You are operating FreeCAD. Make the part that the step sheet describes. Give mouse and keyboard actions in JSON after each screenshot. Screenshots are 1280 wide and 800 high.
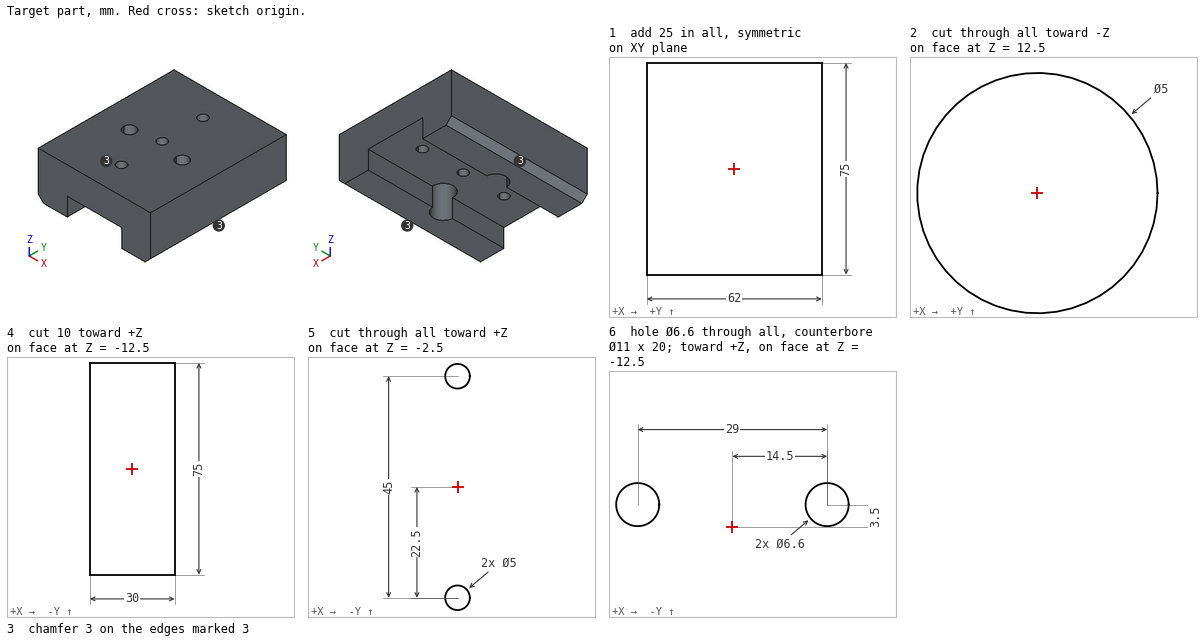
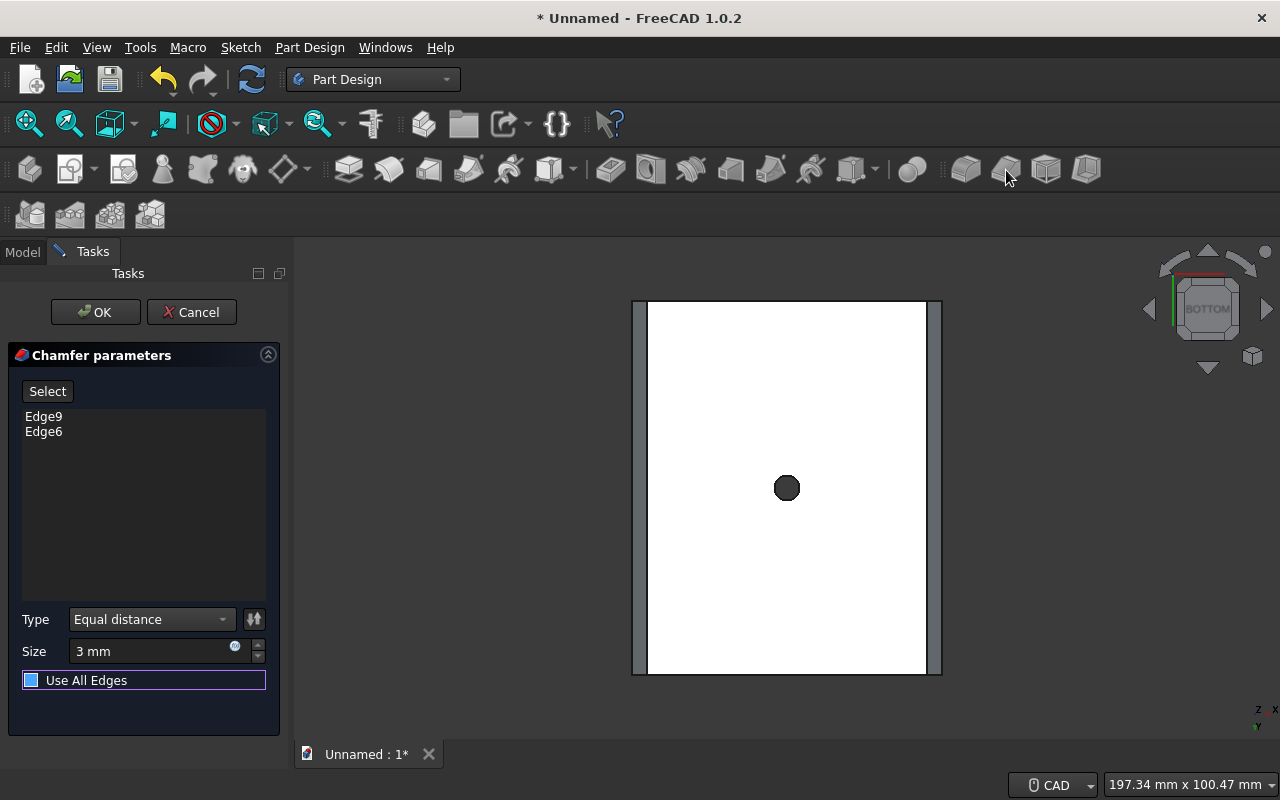
{"action": "left_click", "coordinate": [96, 312]}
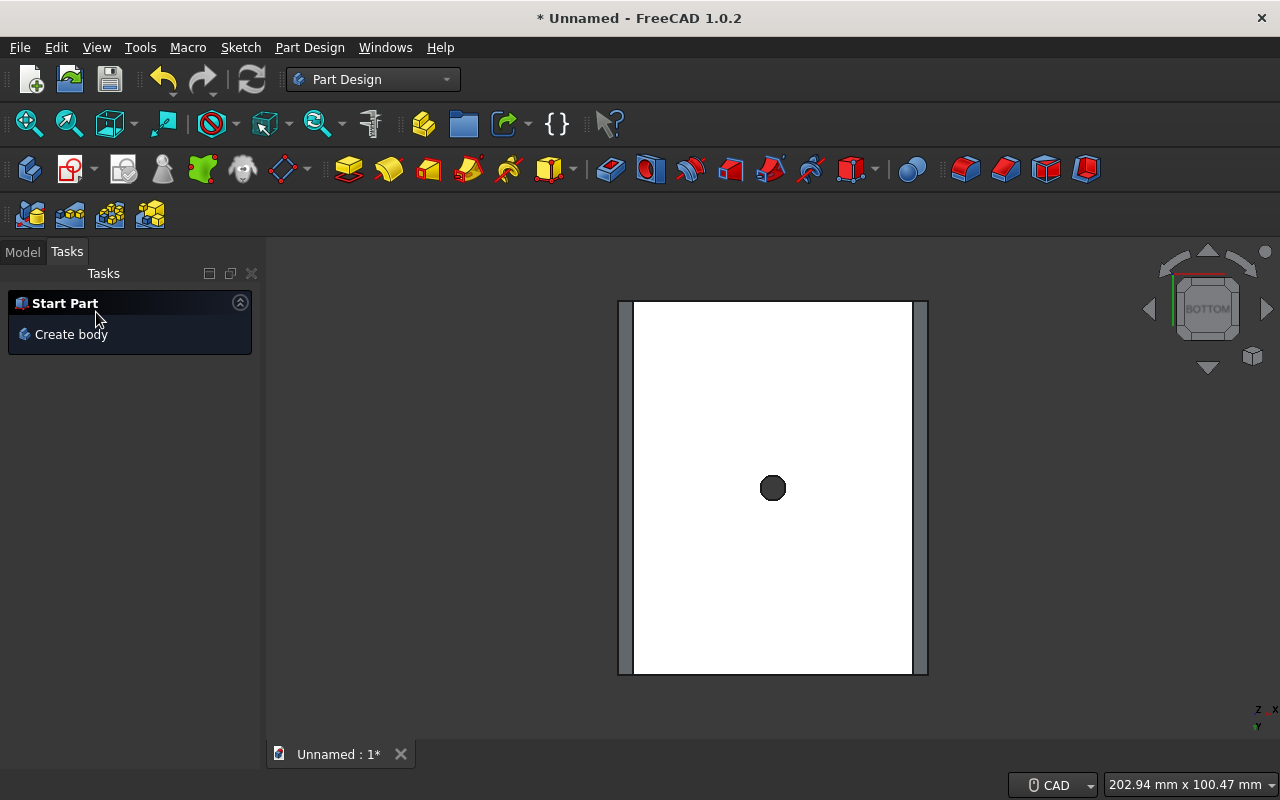
{"action": "left_click", "coordinate": [813, 380]}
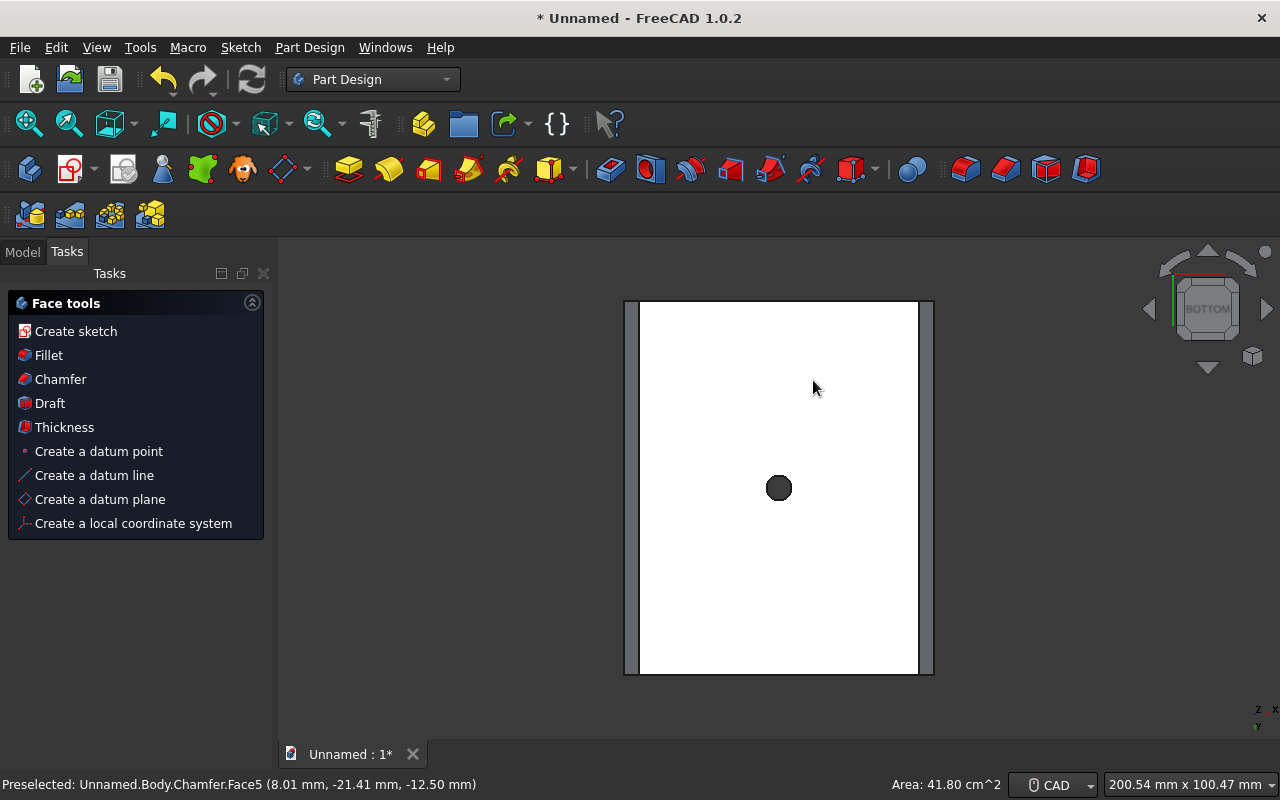
{"action": "left_click", "coordinate": [70, 170]}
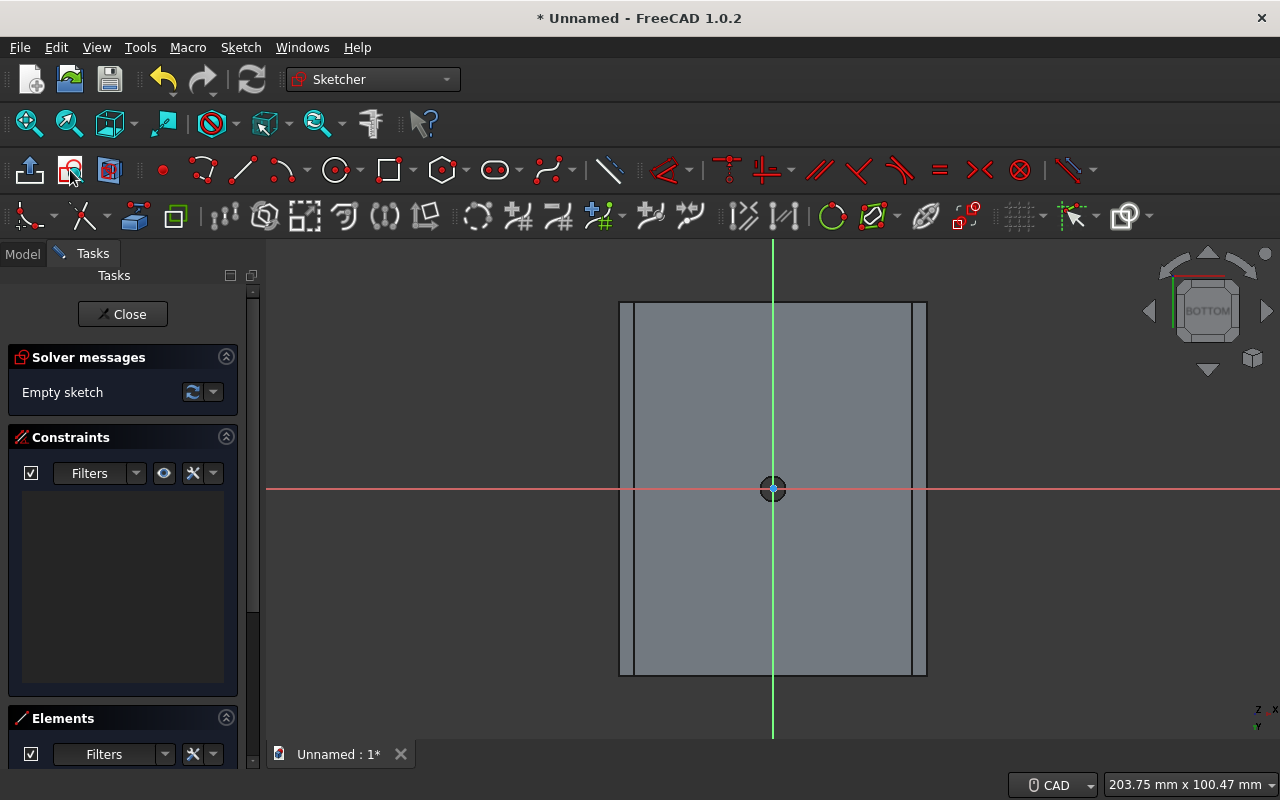
{"action": "key", "text": "g v"}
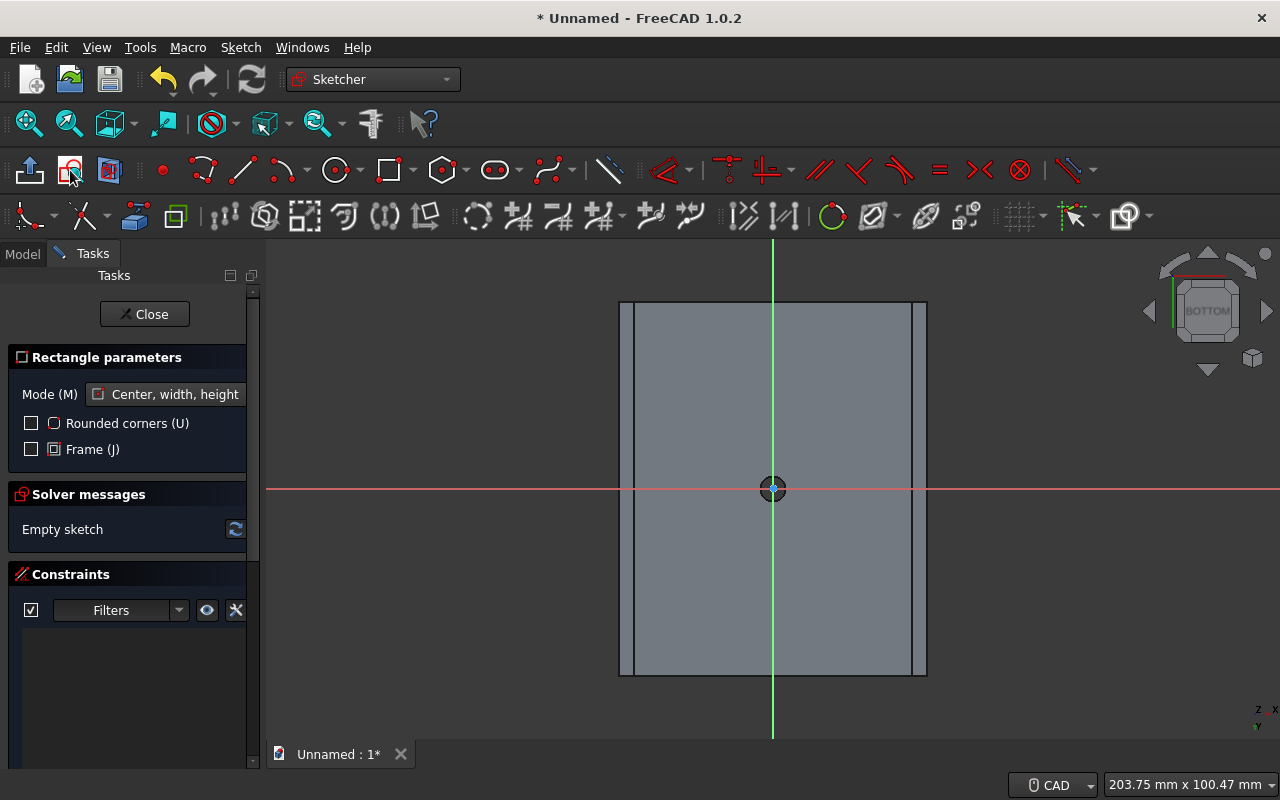
{"action": "left_click", "coordinate": [773, 489]}
{"action": "left_click", "coordinate": [848, 302]}
{"action": "key", "text": "Escape"}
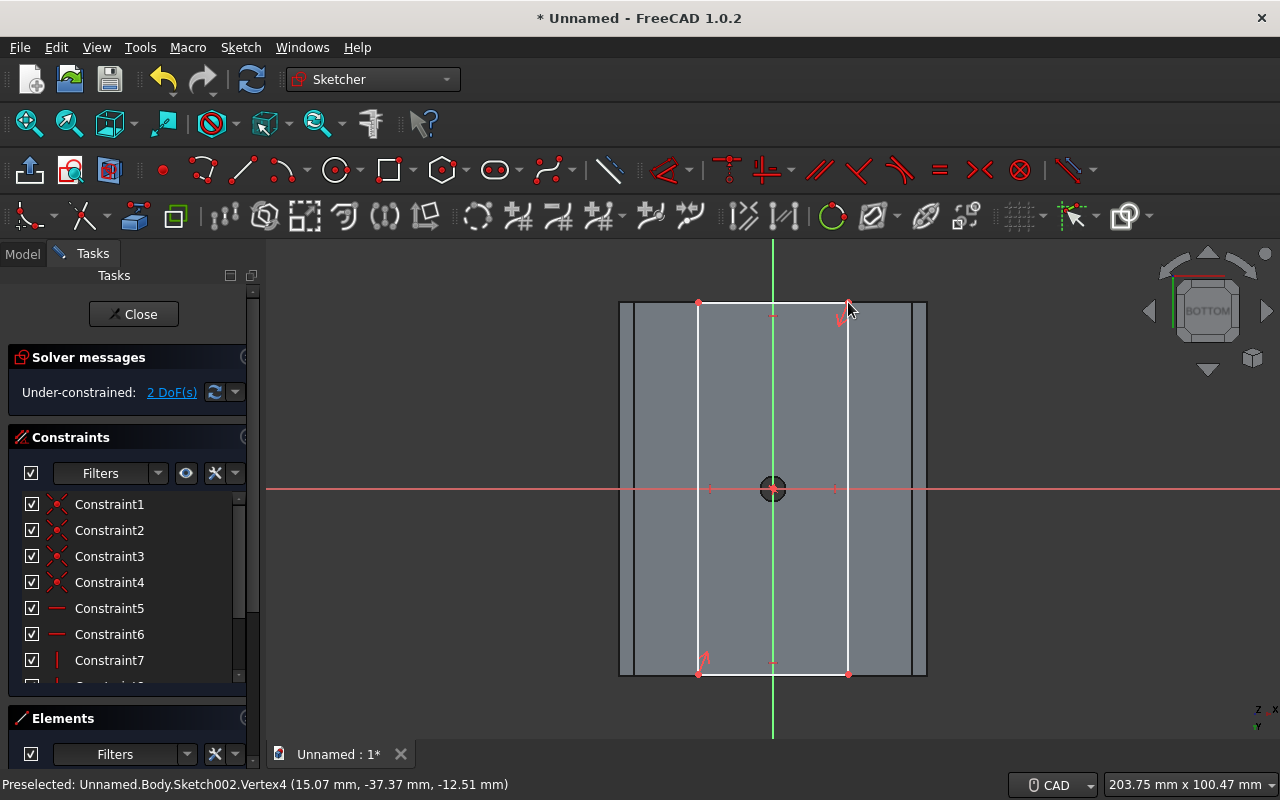
{"action": "key", "text": "d"}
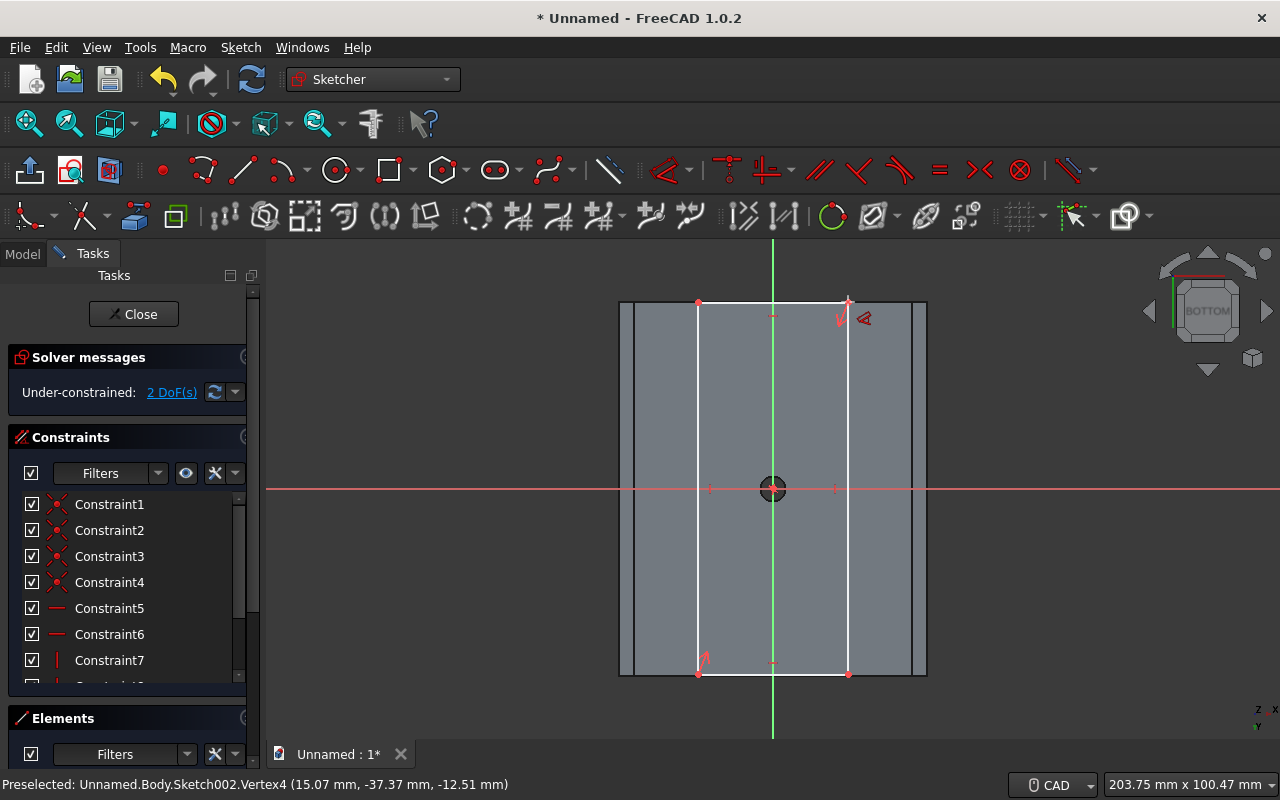
{"action": "left_click", "coordinate": [743, 675]}
{"action": "left_click", "coordinate": [739, 709]}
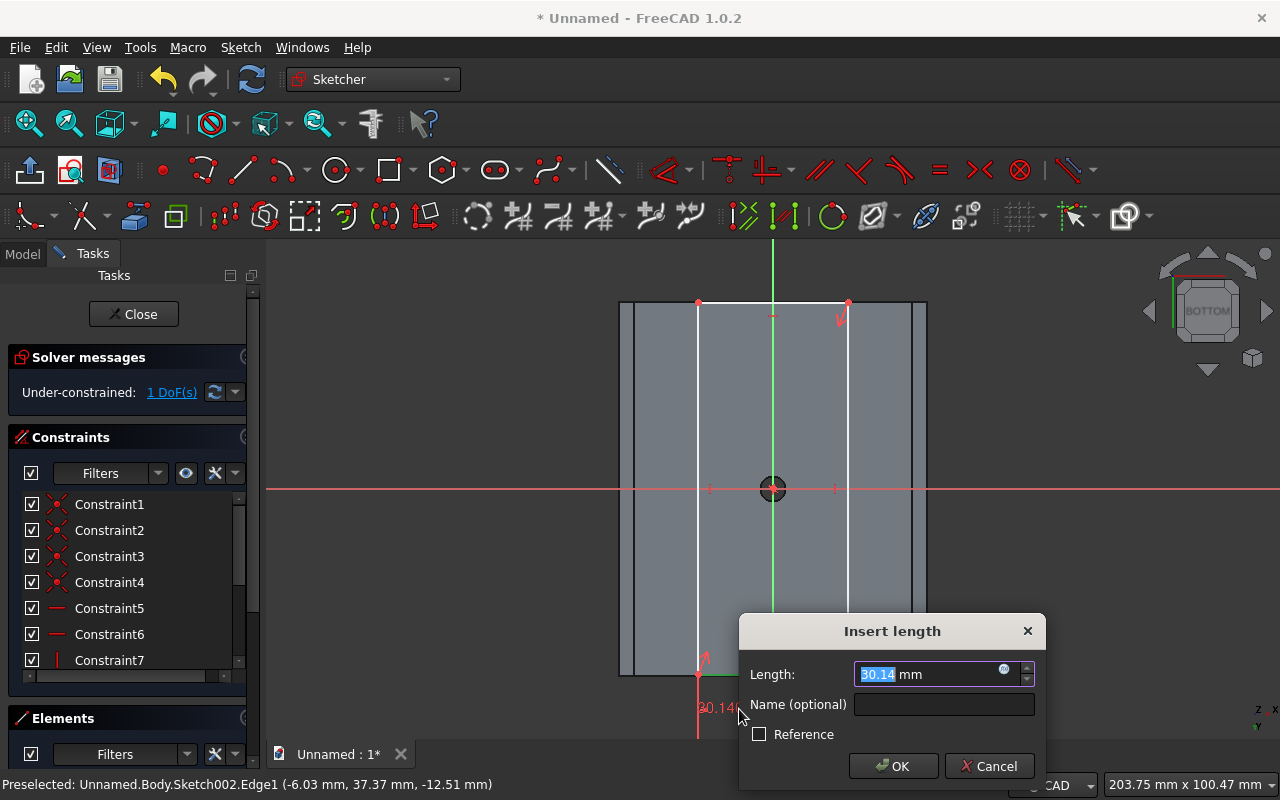
{"action": "type", "text": "30"}
{"action": "key", "text": "Return"}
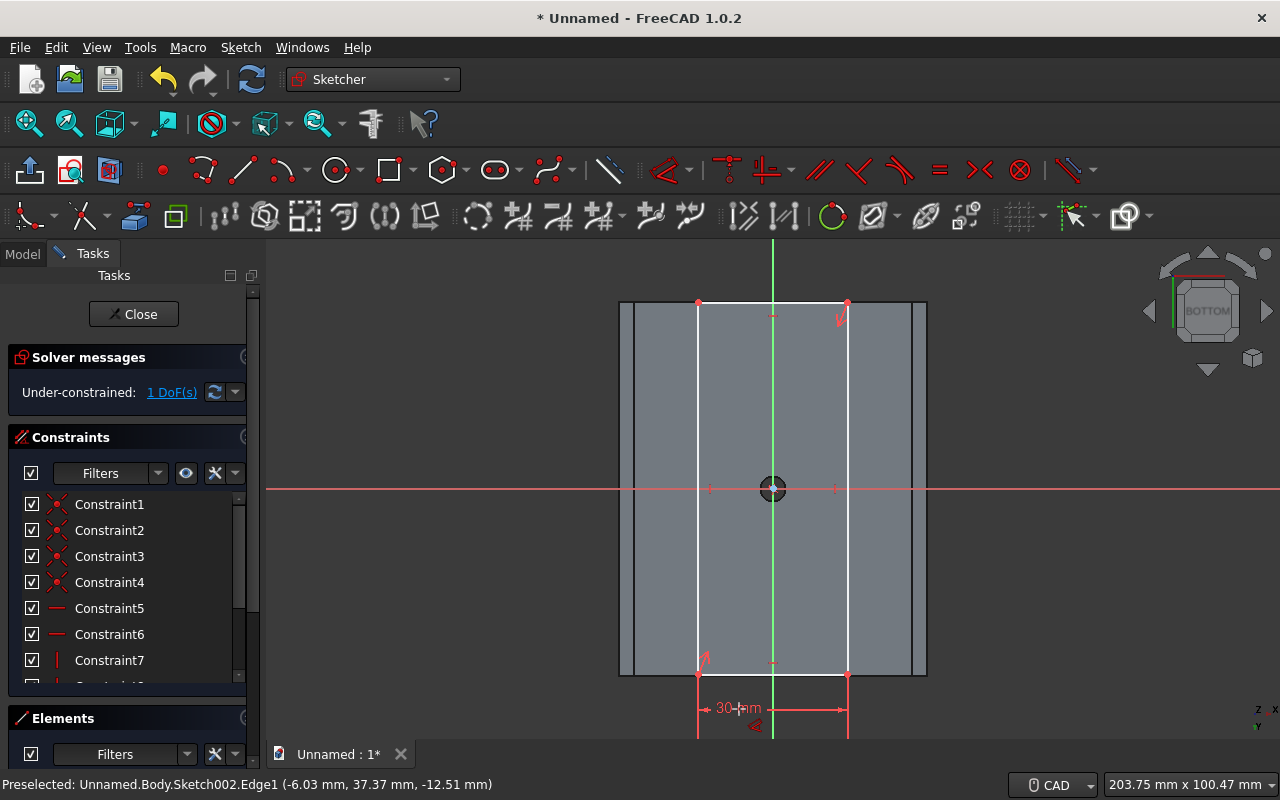
{"action": "left_click", "coordinate": [848, 563]}
{"action": "left_click", "coordinate": [882, 403]}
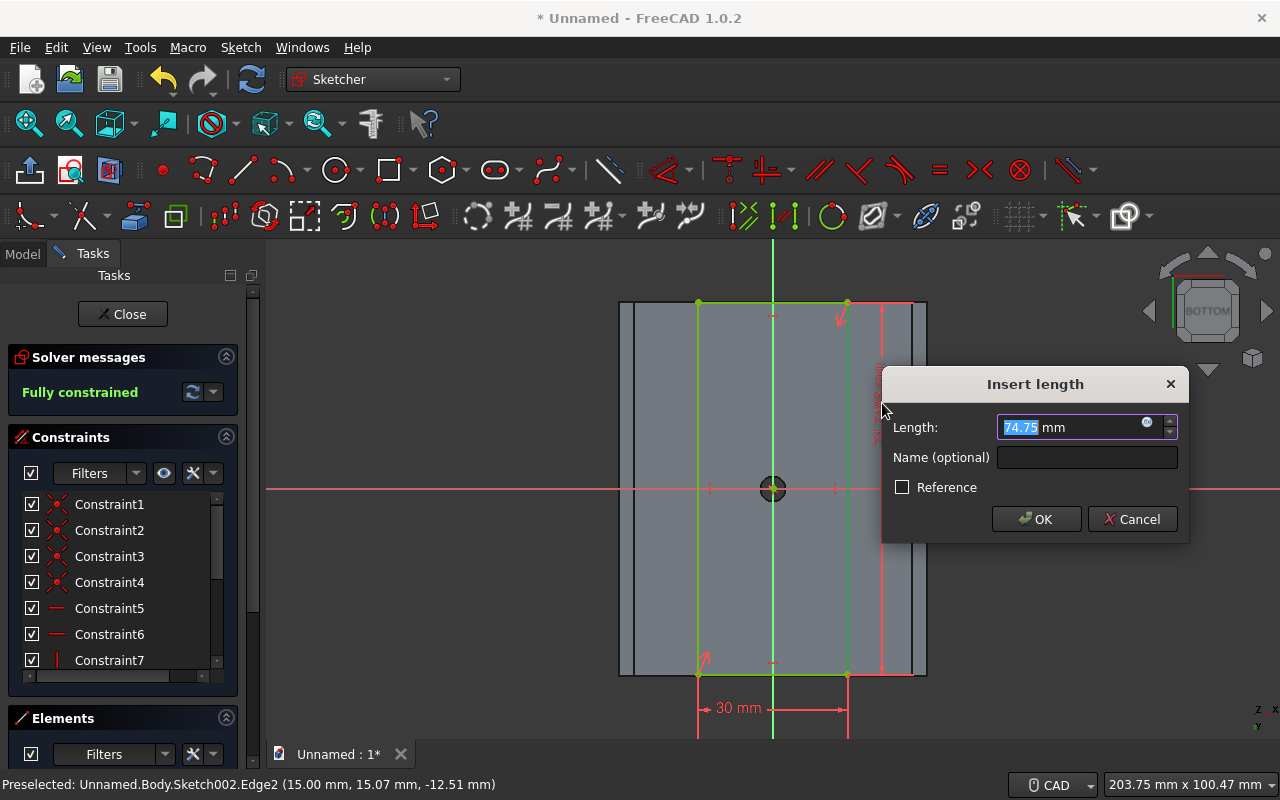
{"action": "type", "text": "75"}
{"action": "key", "text": "Return"}
{"action": "key", "text": "Escape"}